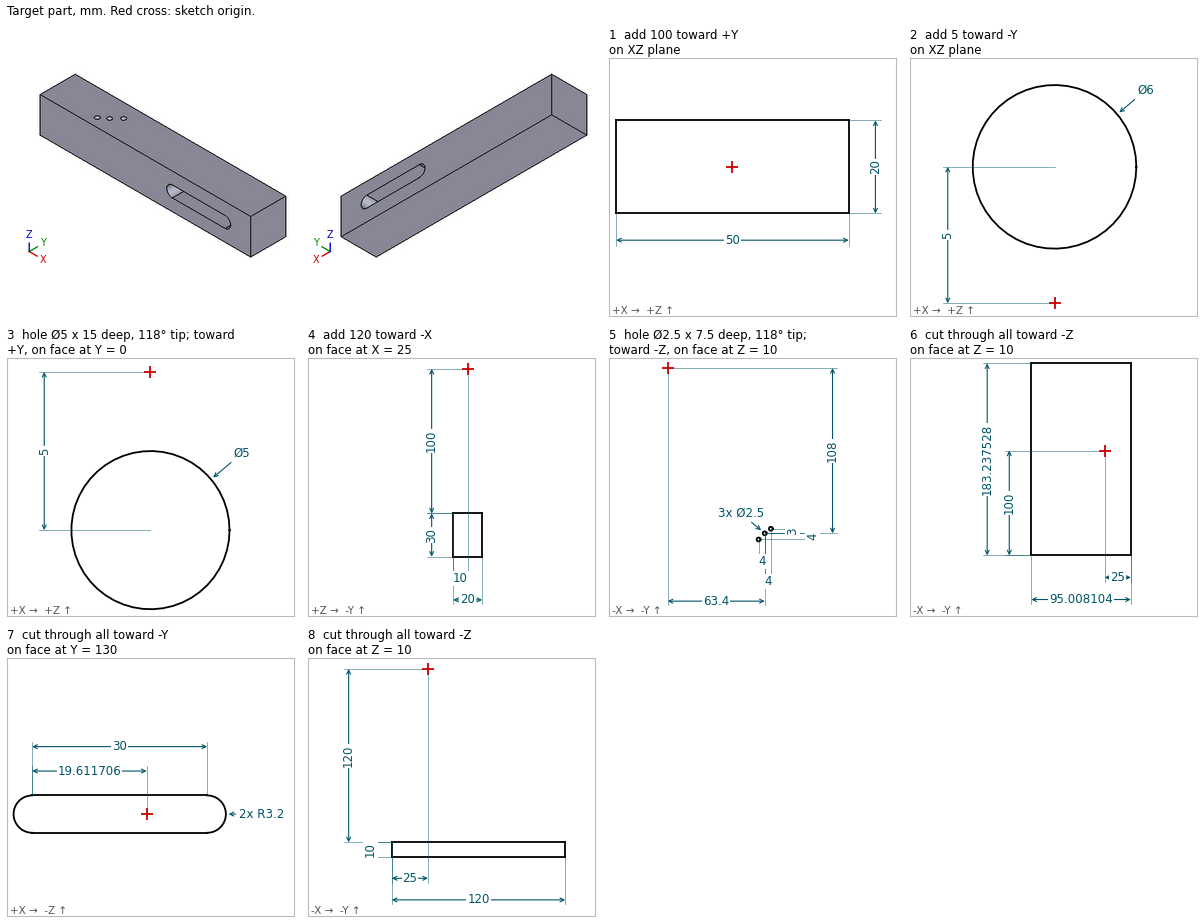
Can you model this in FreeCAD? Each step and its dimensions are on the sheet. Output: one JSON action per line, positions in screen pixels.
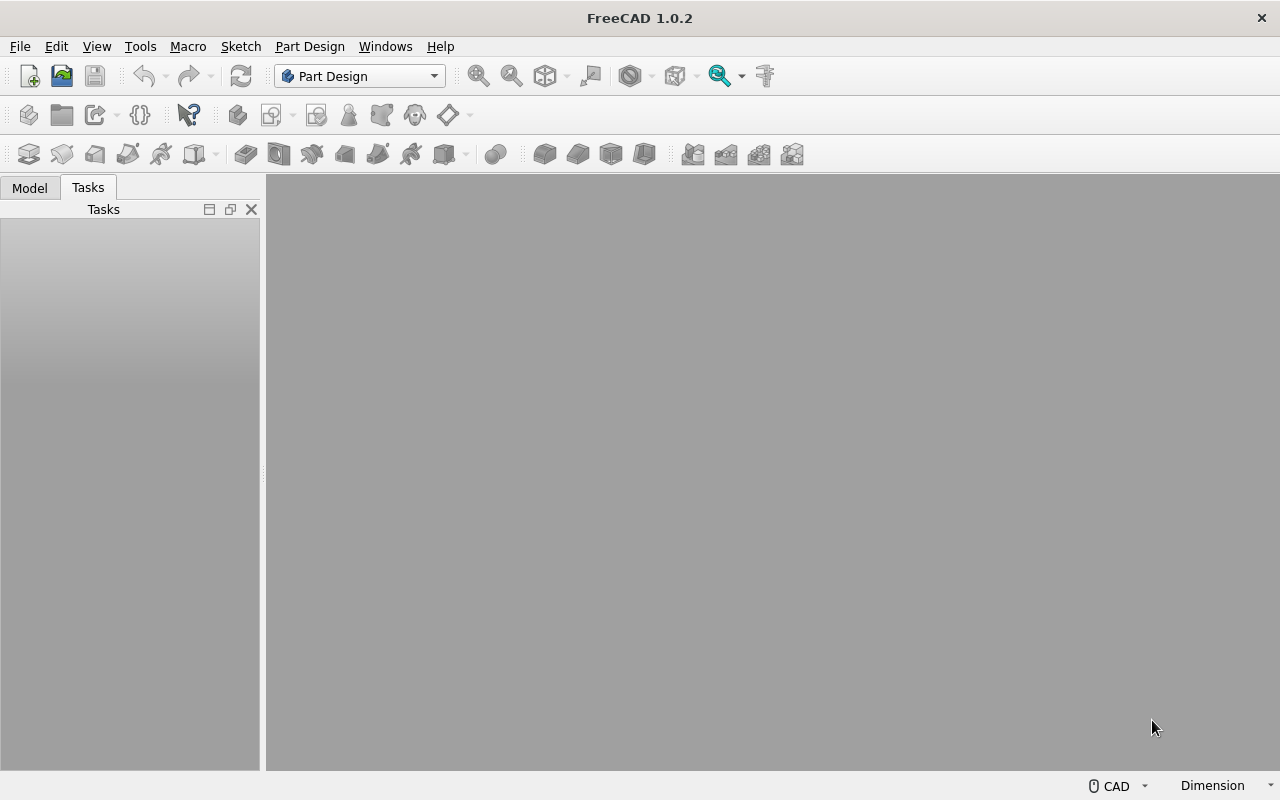
{"action": "left_click", "coordinate": [29, 76]}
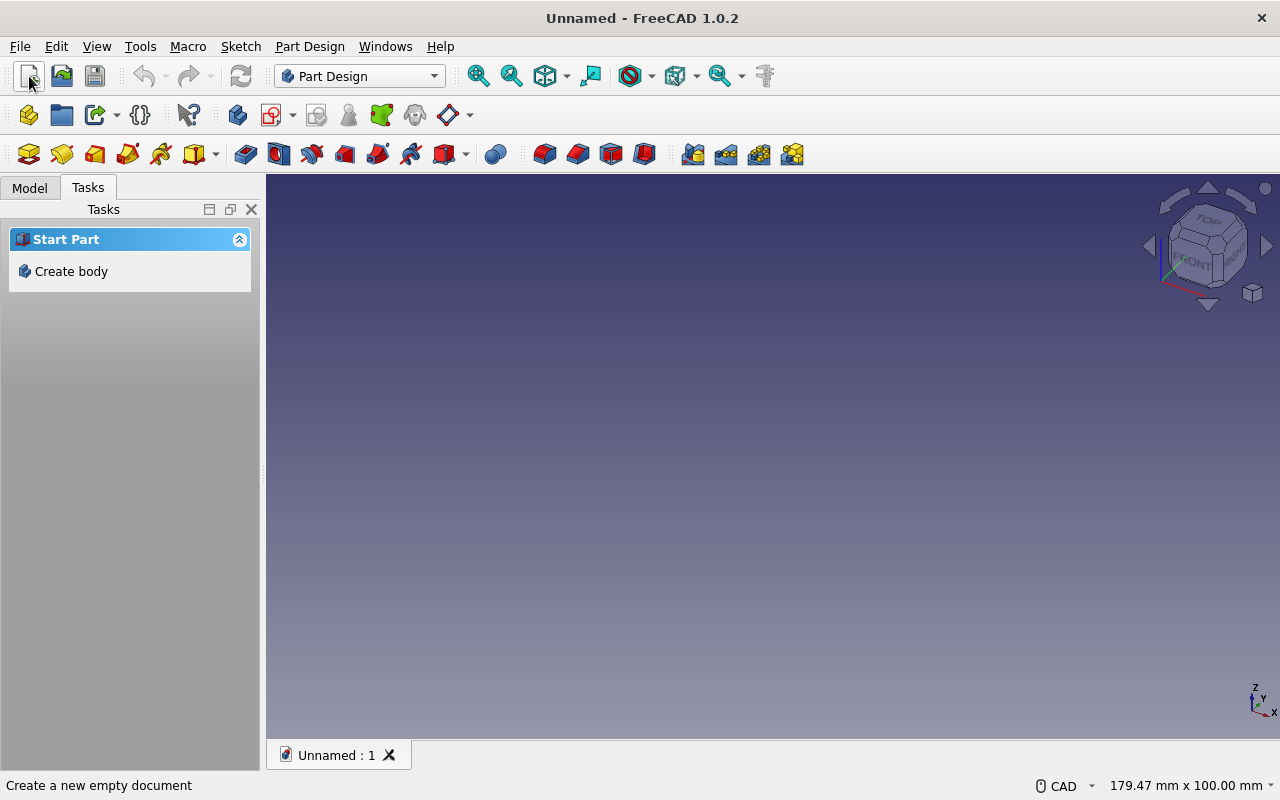
{"action": "left_click", "coordinate": [270, 116]}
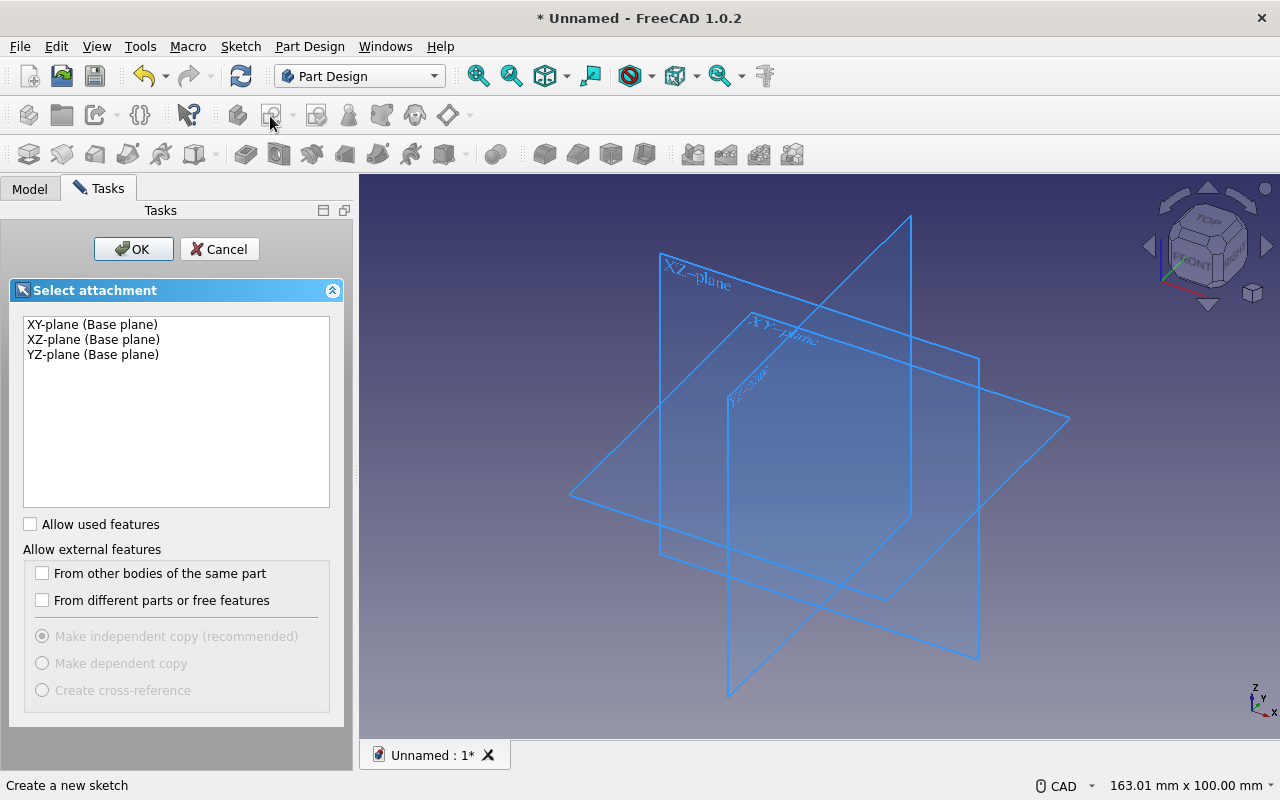
{"action": "left_click", "coordinate": [84, 340]}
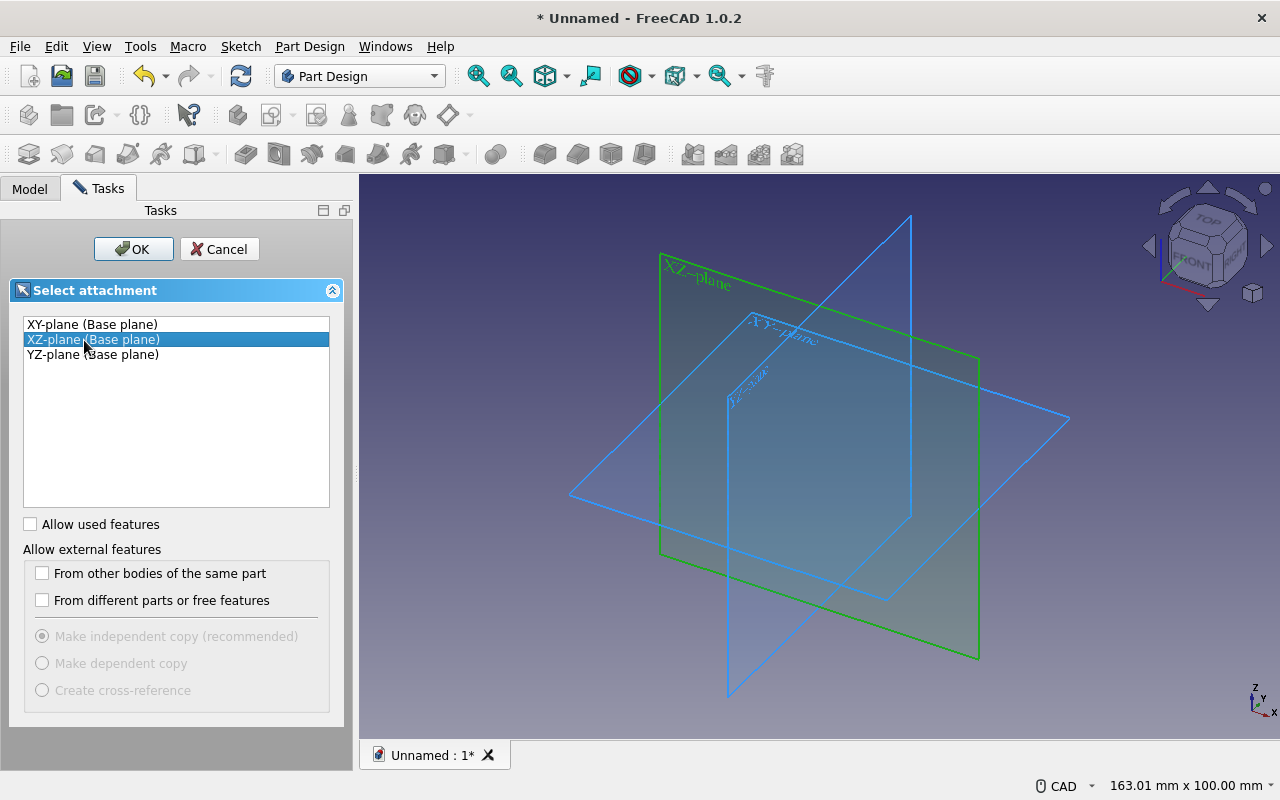
{"action": "left_click", "coordinate": [134, 249]}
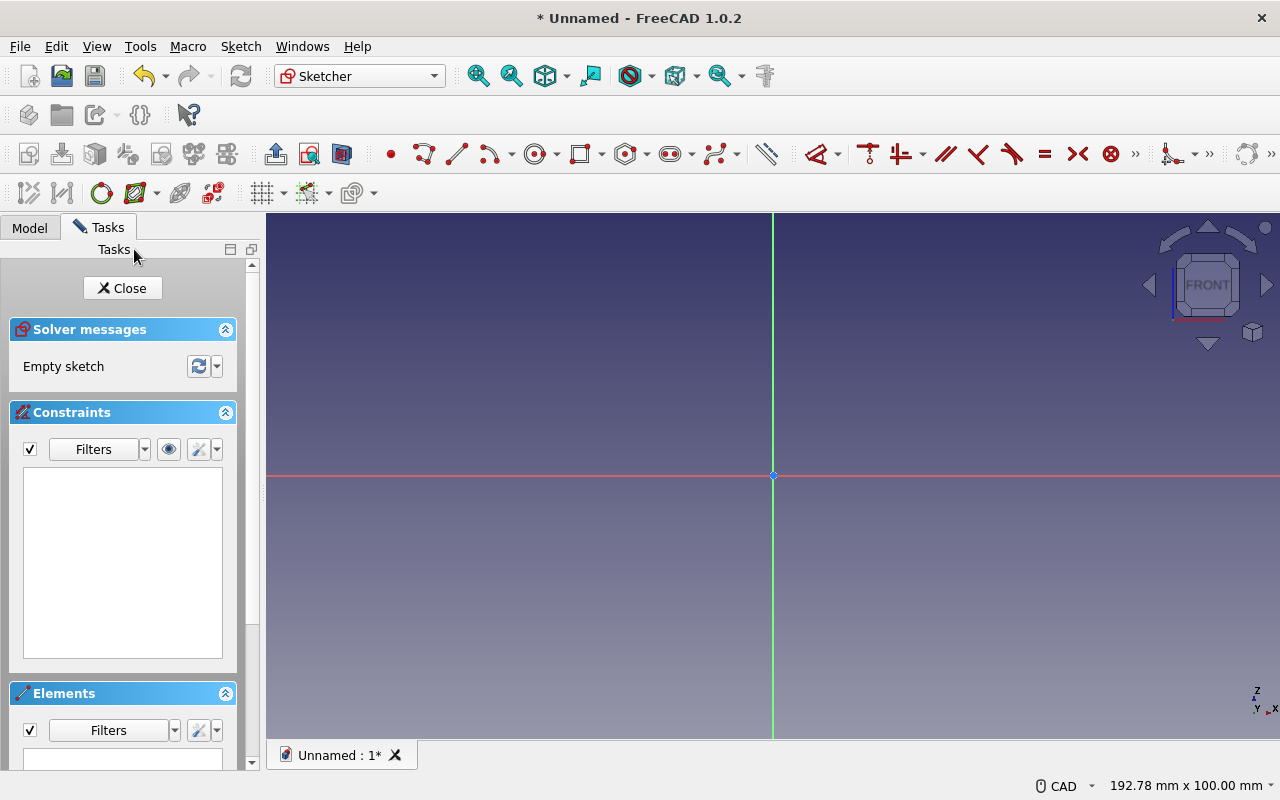
{"action": "scroll", "coordinate": [829, 476], "scroll_direction": "up", "scroll_amount": 4}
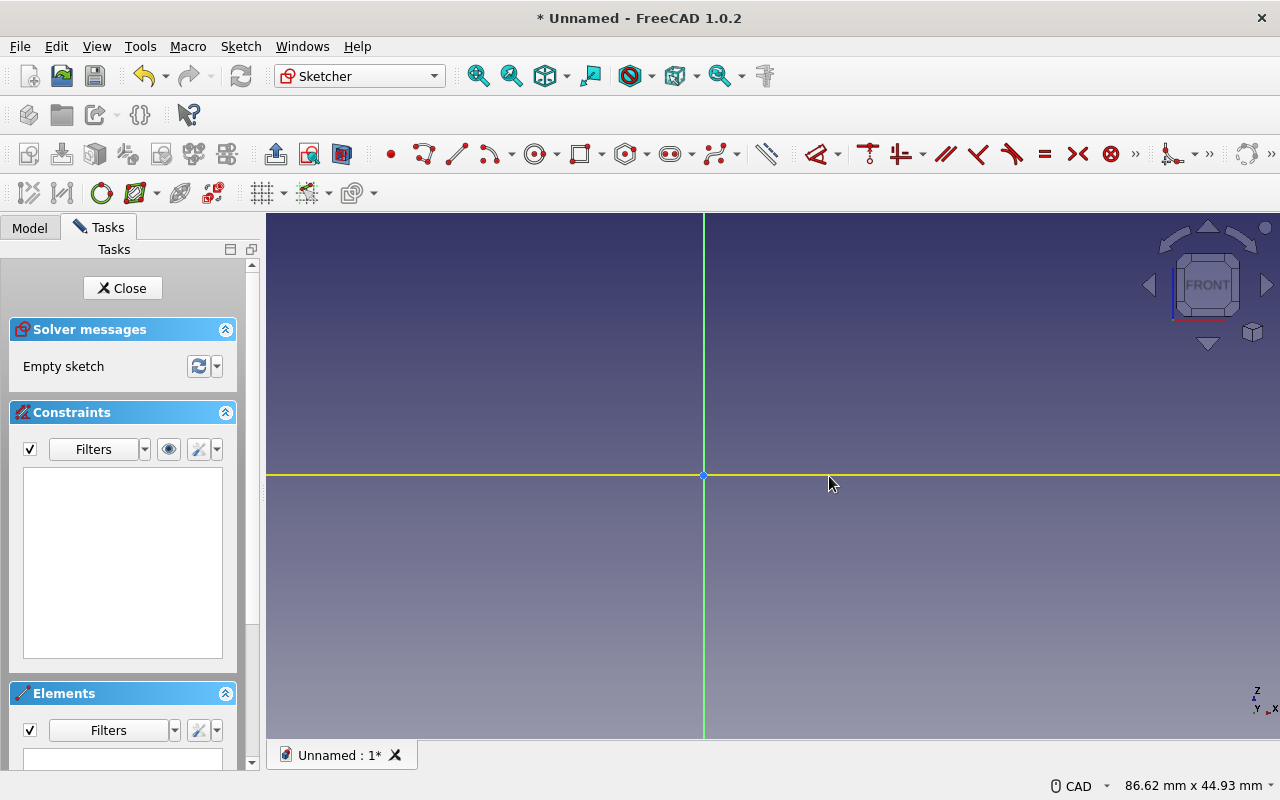
{"action": "key", "text": "g v"}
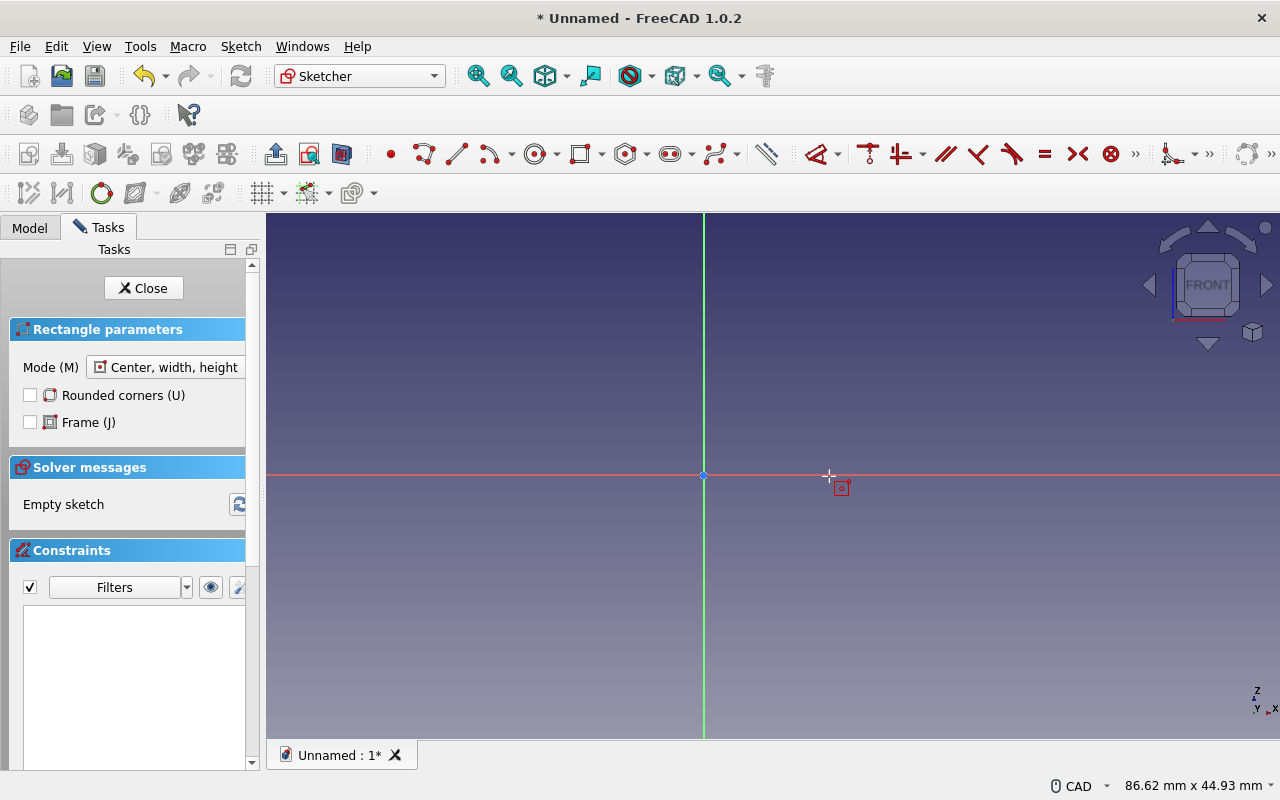
{"action": "left_click", "coordinate": [704, 475]}
{"action": "left_click", "coordinate": [996, 358]}
{"action": "key", "text": "Escape"}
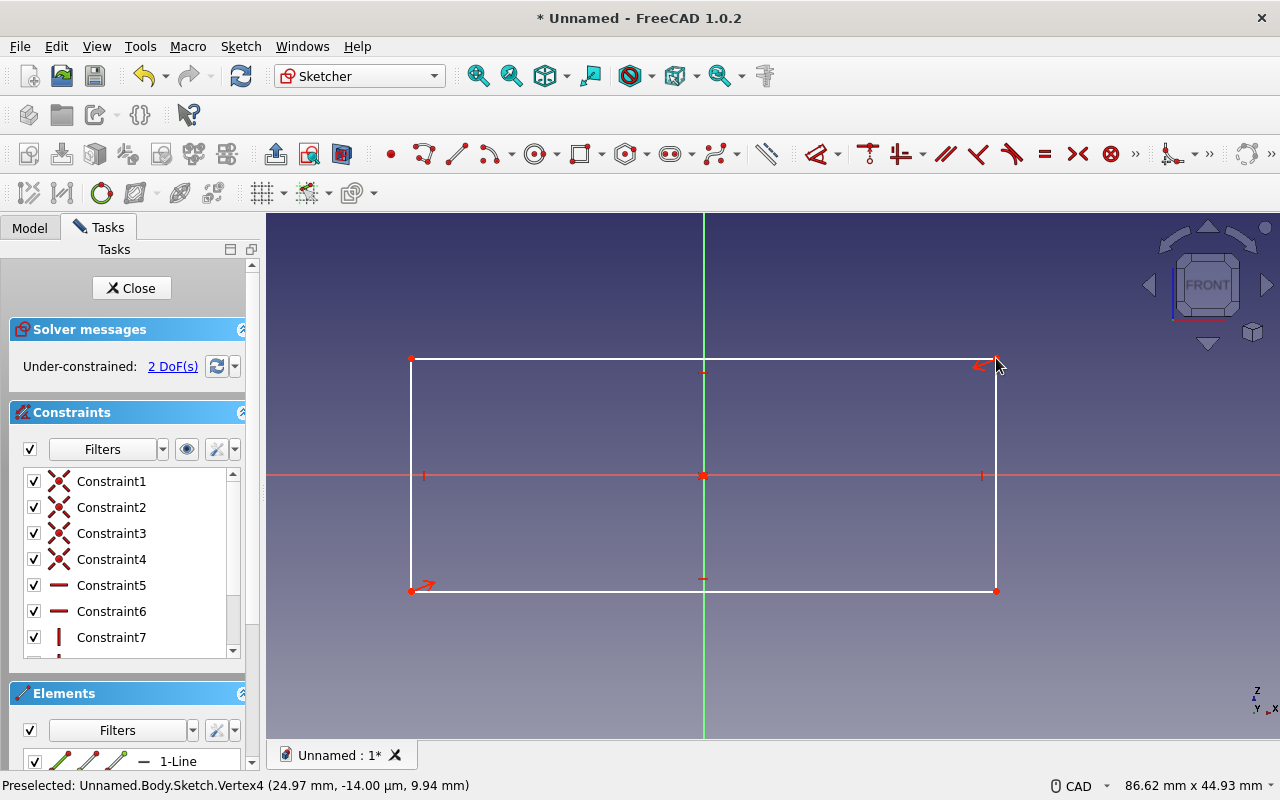
{"action": "left_click", "coordinate": [816, 154]}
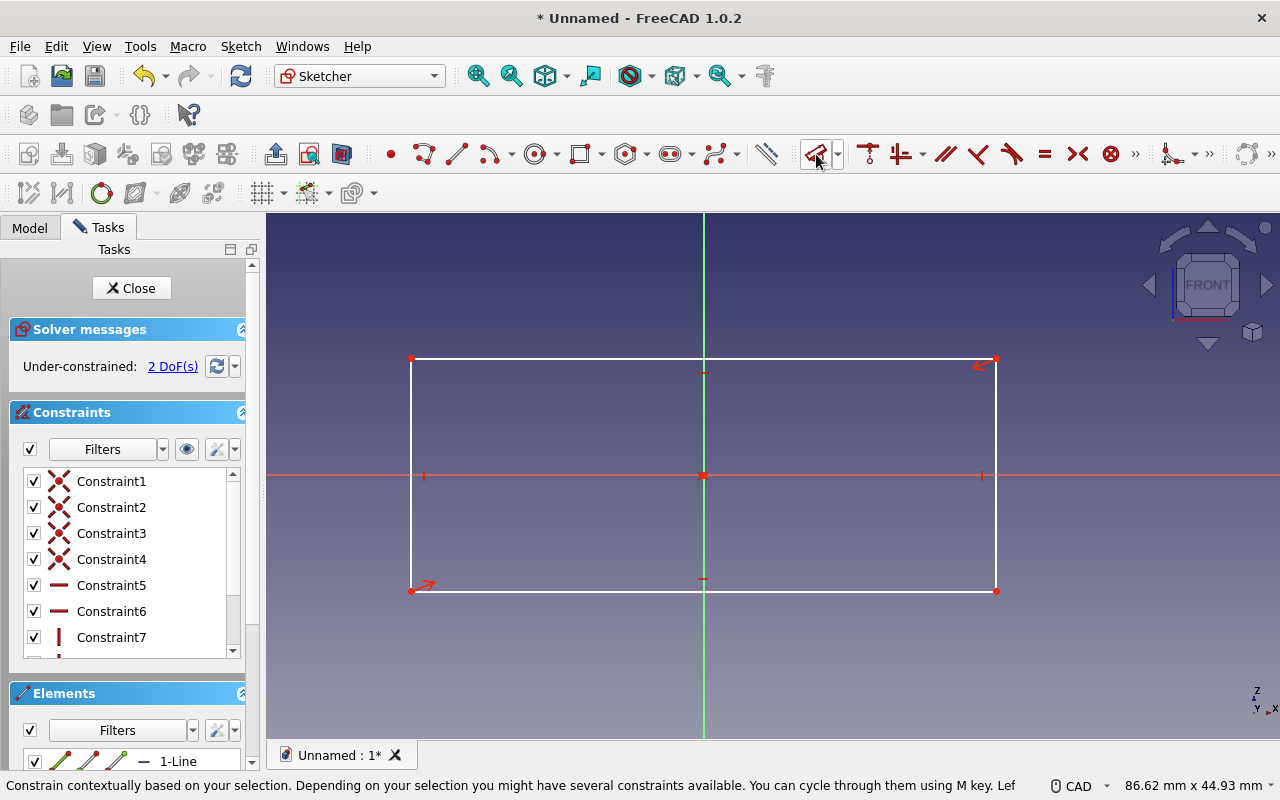
{"action": "left_click", "coordinate": [587, 592]}
{"action": "left_click", "coordinate": [569, 626]}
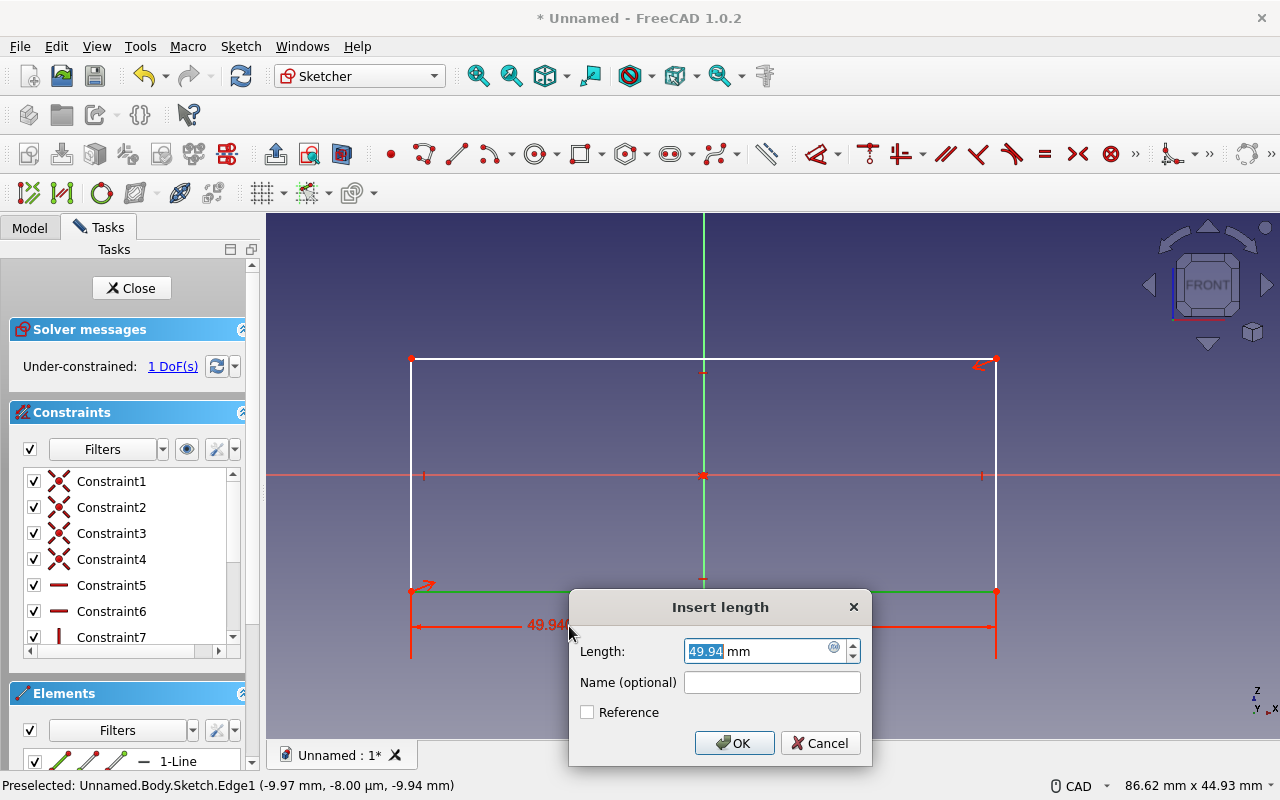
{"action": "type", "text": "50"}
{"action": "key", "text": "Return"}